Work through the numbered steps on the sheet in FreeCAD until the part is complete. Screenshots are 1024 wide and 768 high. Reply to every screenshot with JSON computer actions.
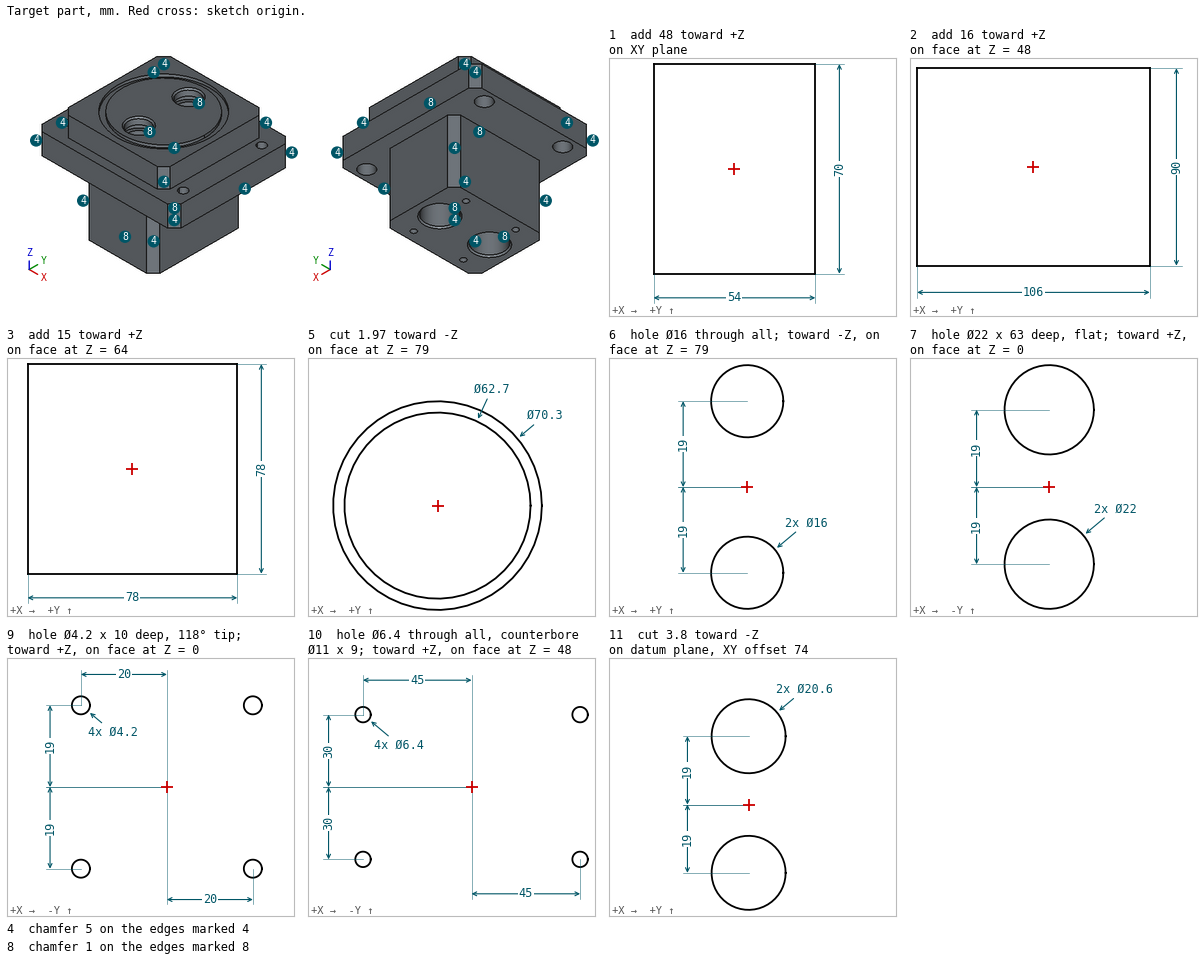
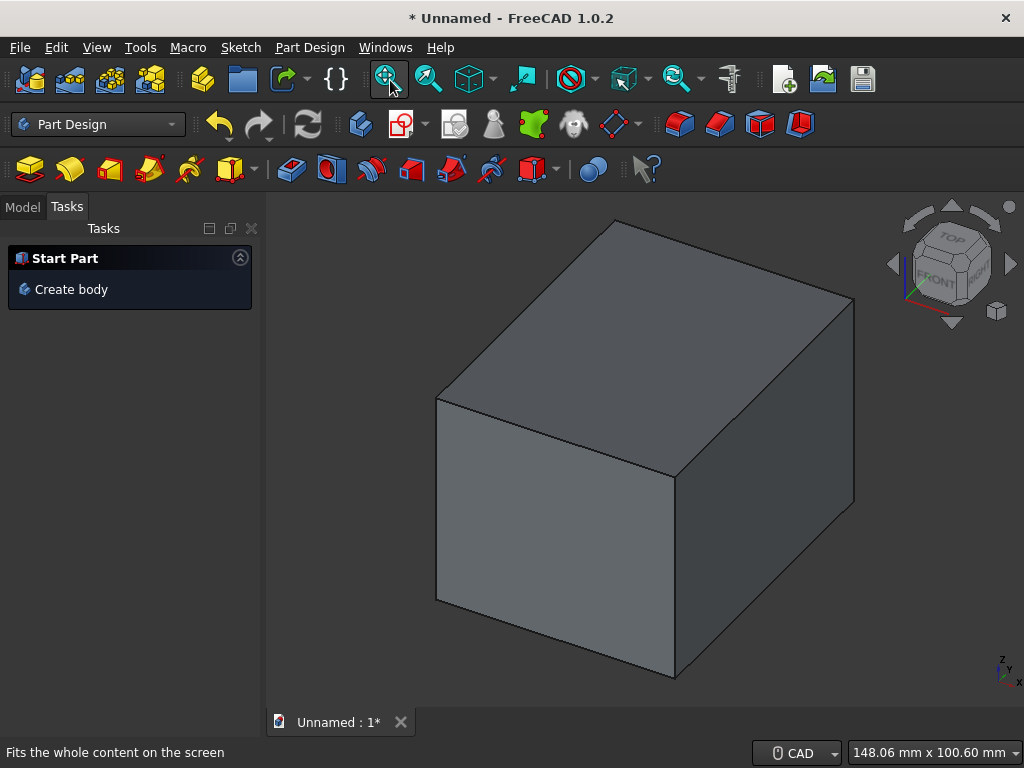
{"action": "left_click", "coordinate": [645, 348]}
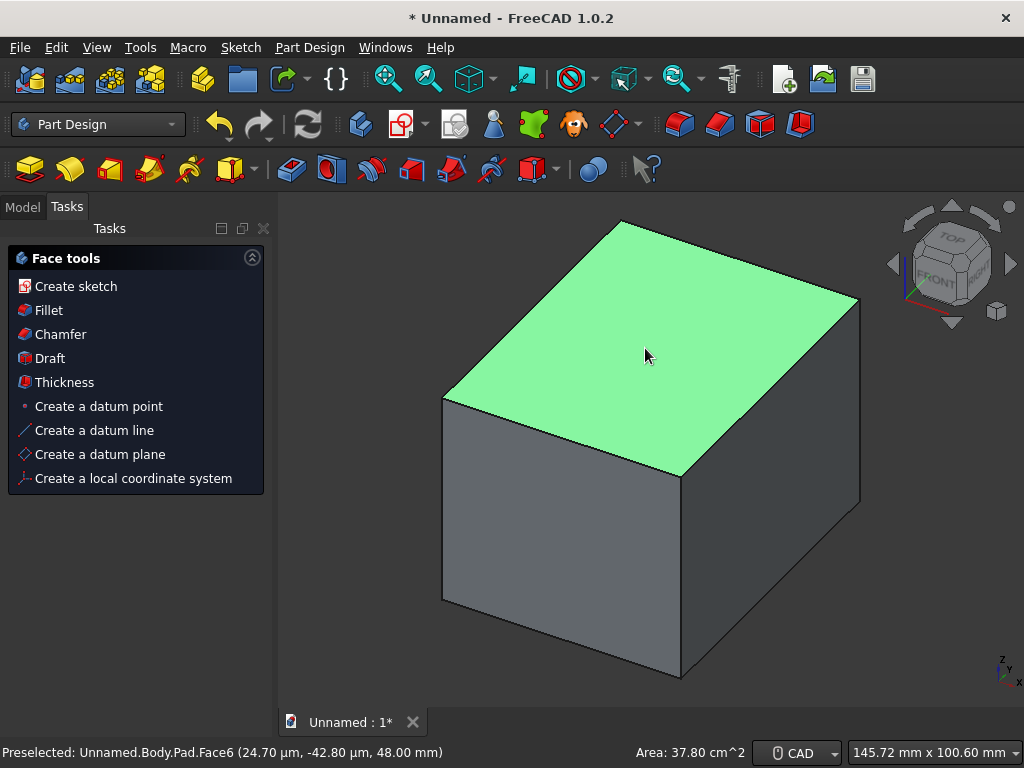
{"action": "left_click", "coordinate": [402, 124]}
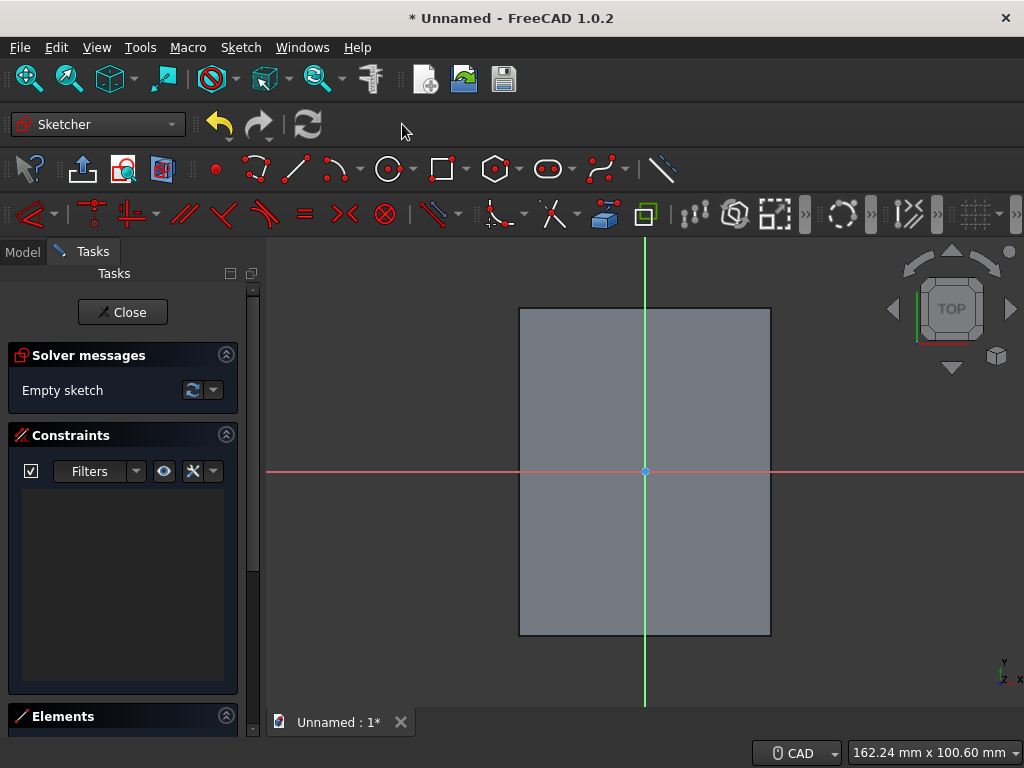
{"action": "scroll", "coordinate": [437, 472], "scroll_direction": "down", "scroll_amount": 2}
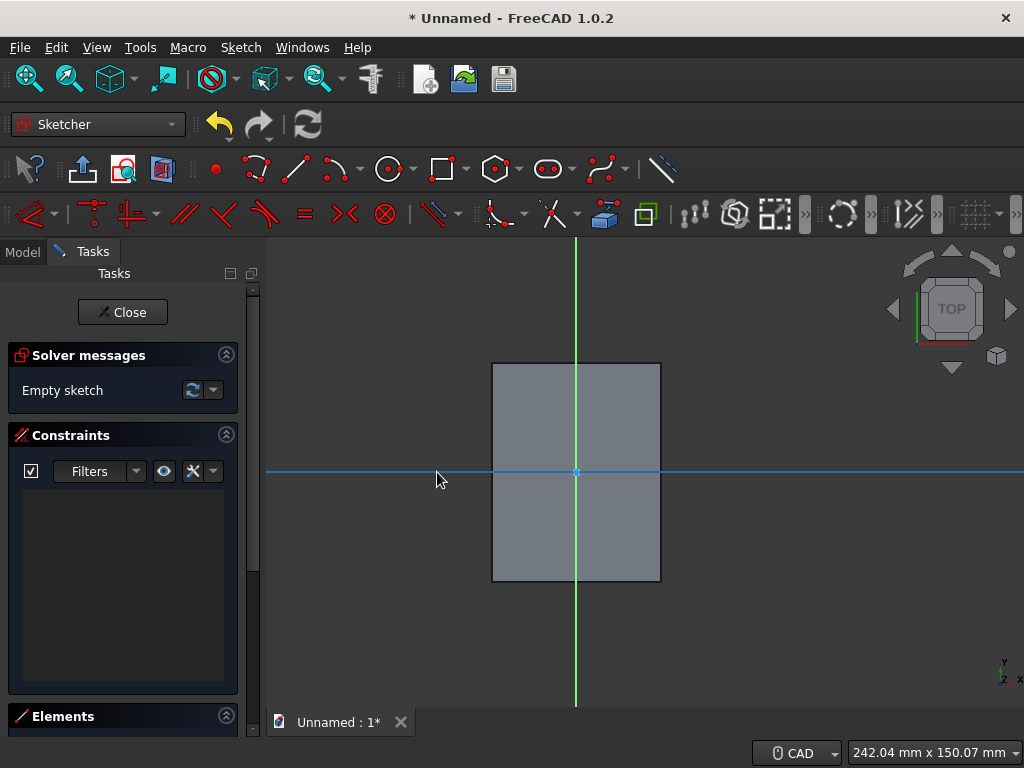
{"action": "left_click", "coordinate": [468, 170]}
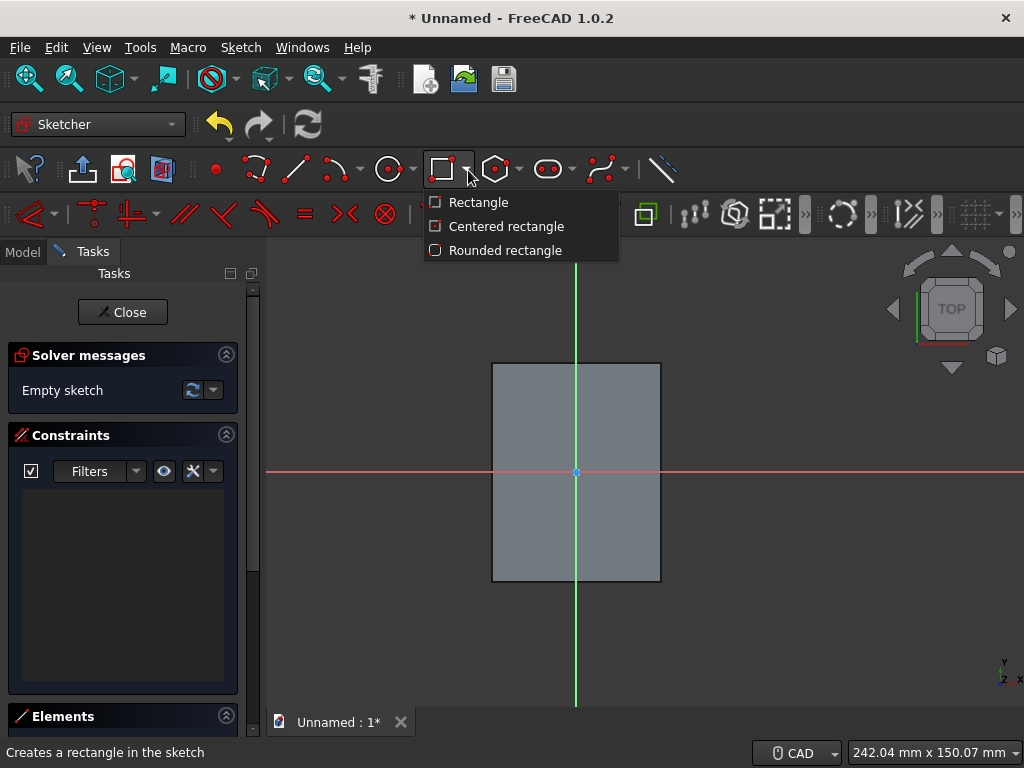
{"action": "left_click", "coordinate": [522, 226]}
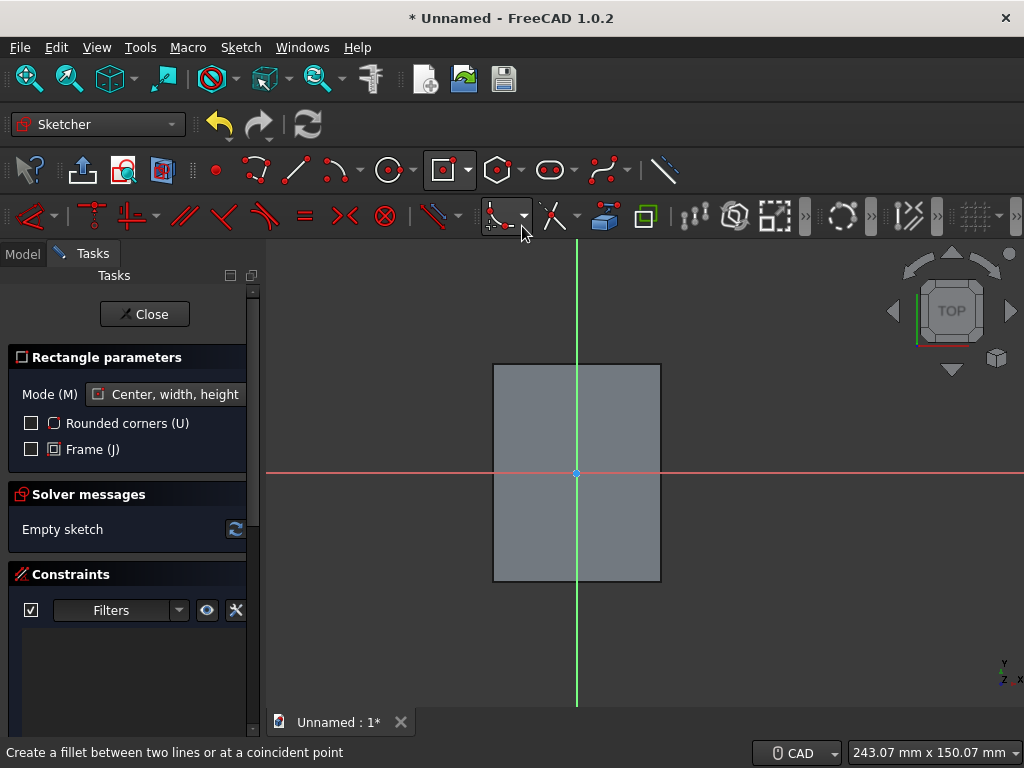
{"action": "left_click", "coordinate": [577, 473]}
{"action": "mouse_move", "coordinate": [742, 333]}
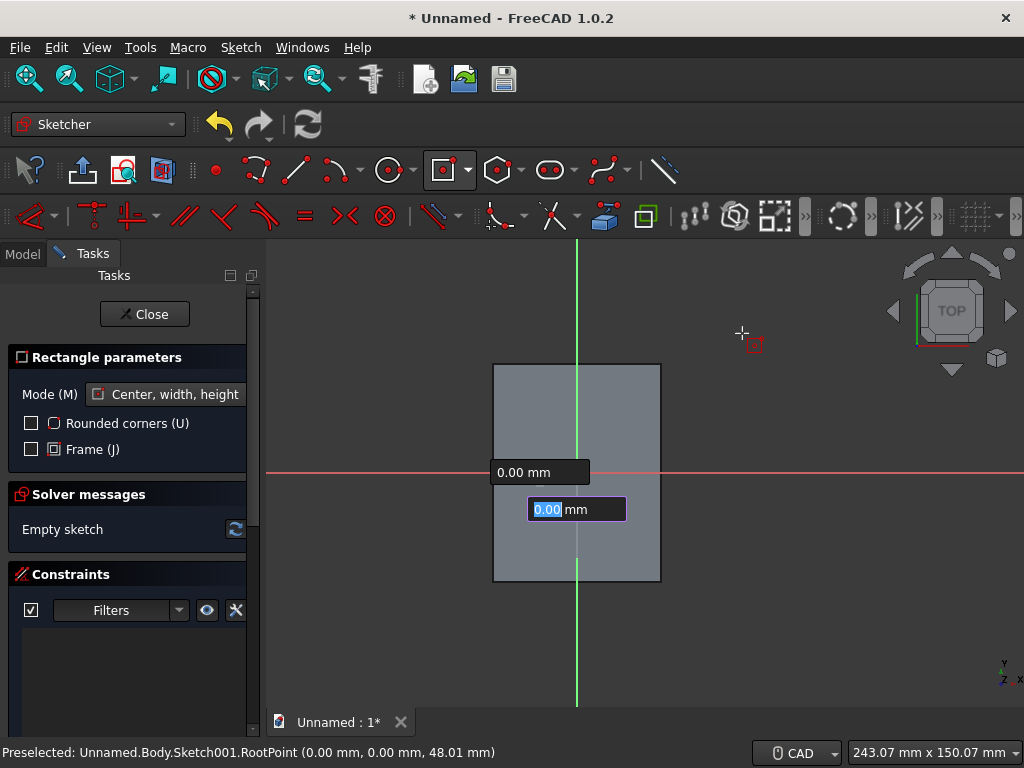
{"action": "type", "text": "106"}
{"action": "key", "text": "Tab"}
{"action": "type", "text": "90"}
{"action": "key", "text": "Return"}
{"action": "key", "text": "Escape"}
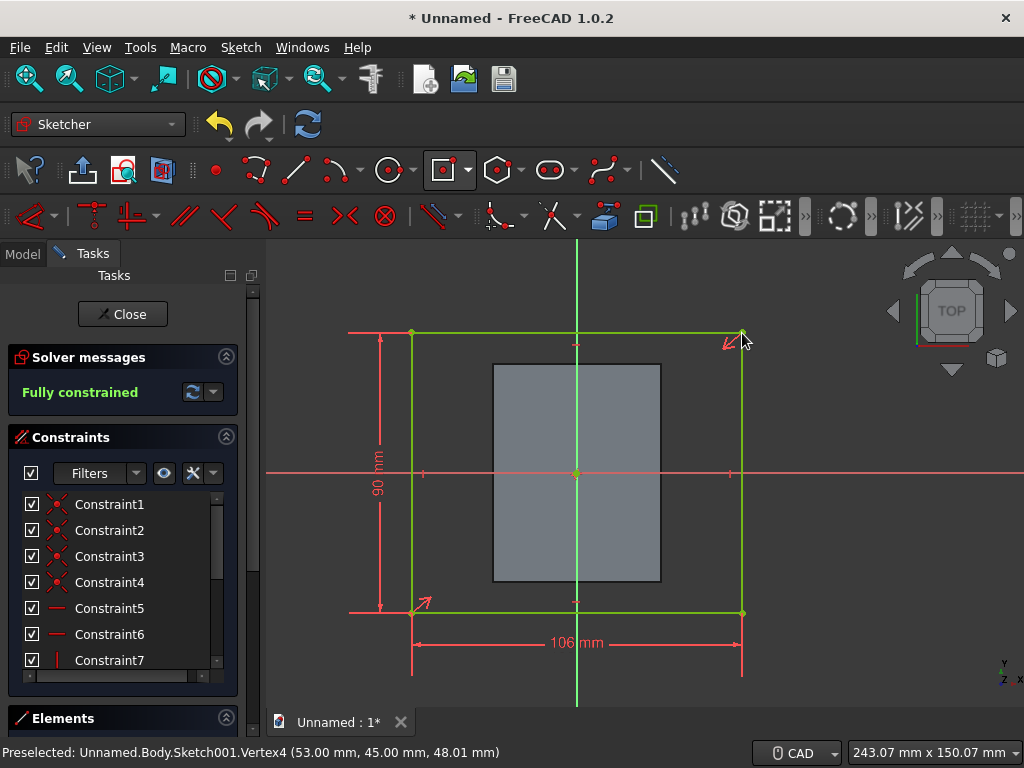
{"action": "left_click", "coordinate": [123, 314]}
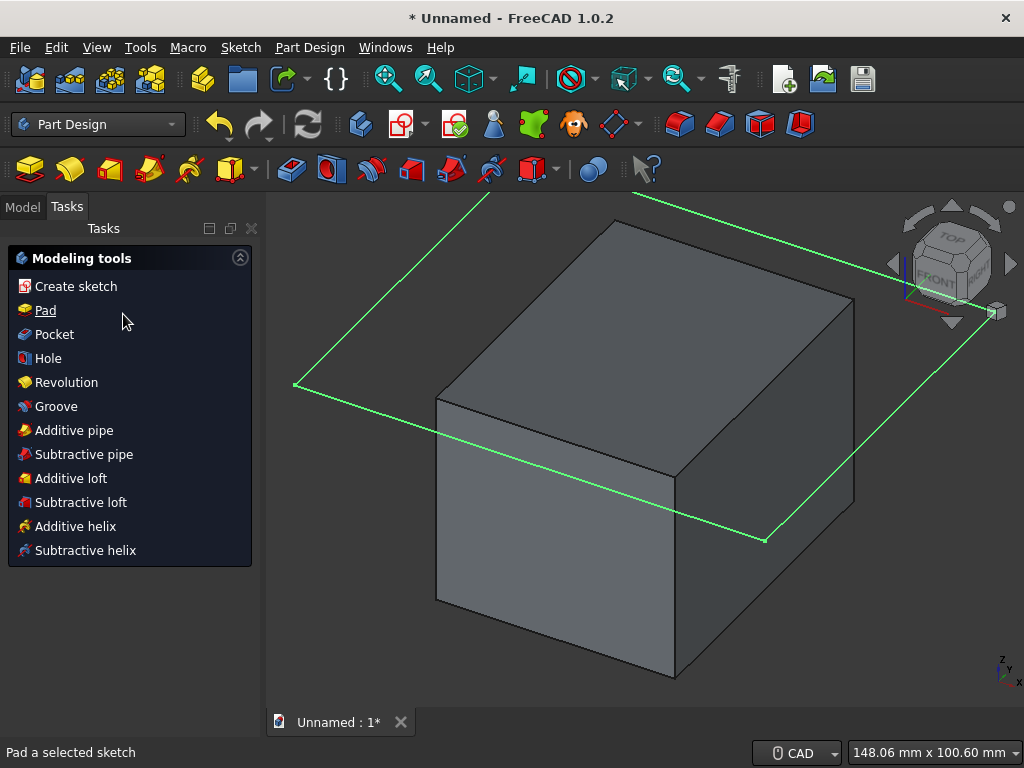
{"action": "left_click", "coordinate": [30, 170]}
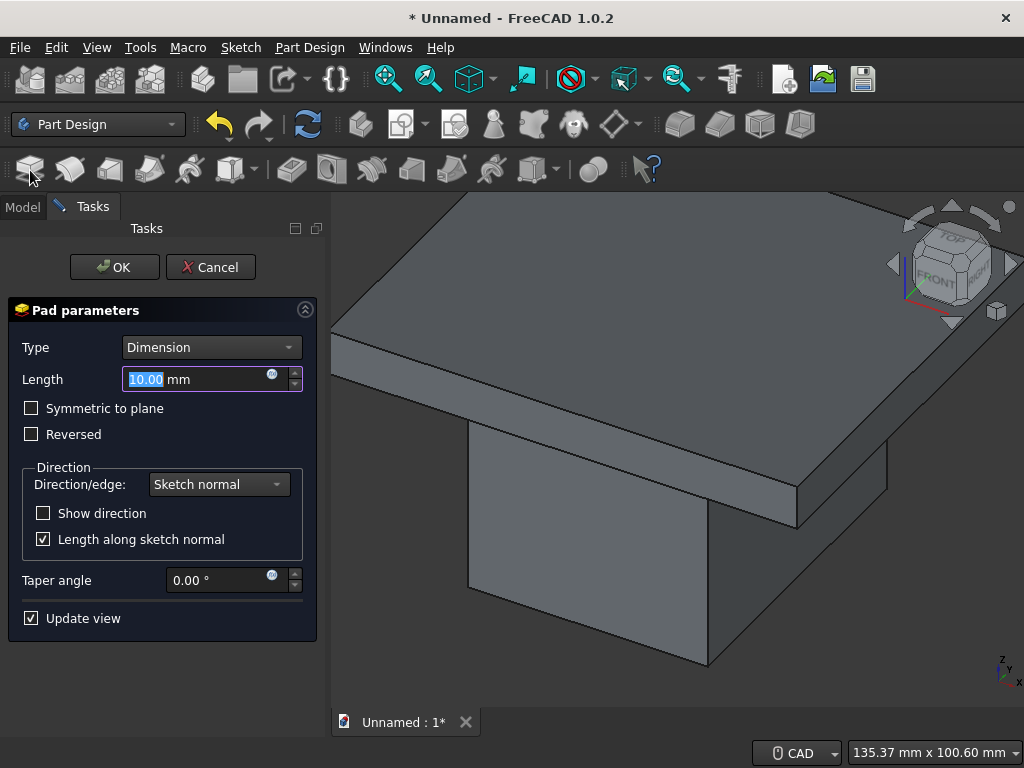
{"action": "type", "text": "16"}
{"action": "key", "text": "Tab"}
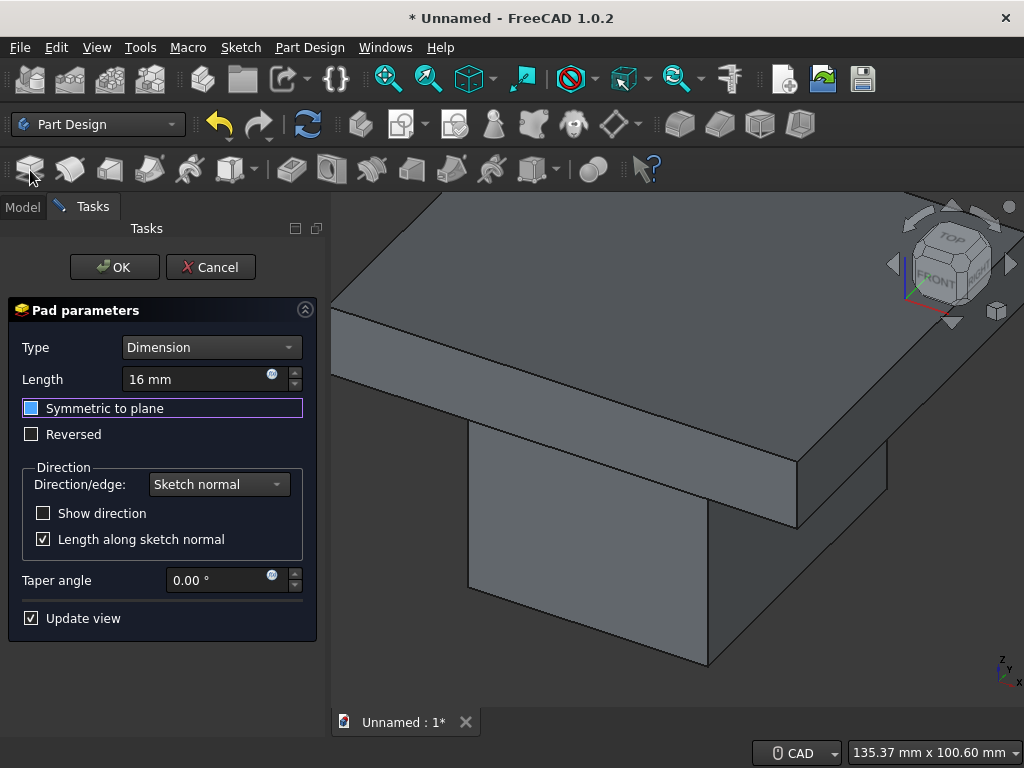
{"action": "left_click", "coordinate": [115, 267]}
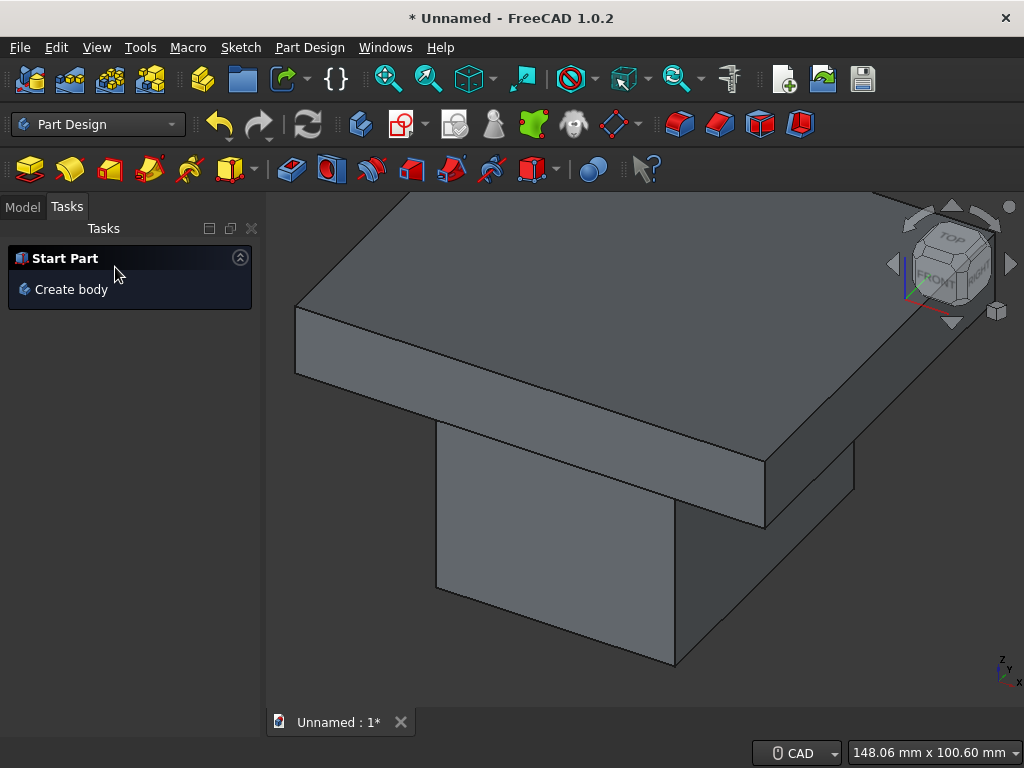
{"action": "left_click", "coordinate": [390, 80]}